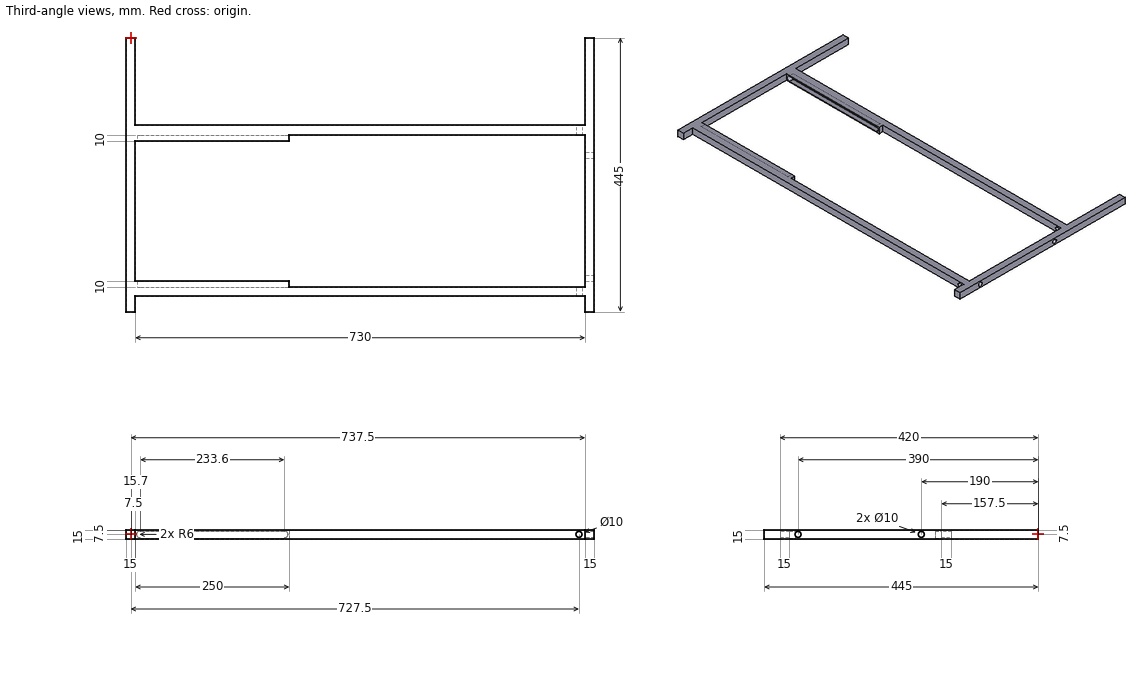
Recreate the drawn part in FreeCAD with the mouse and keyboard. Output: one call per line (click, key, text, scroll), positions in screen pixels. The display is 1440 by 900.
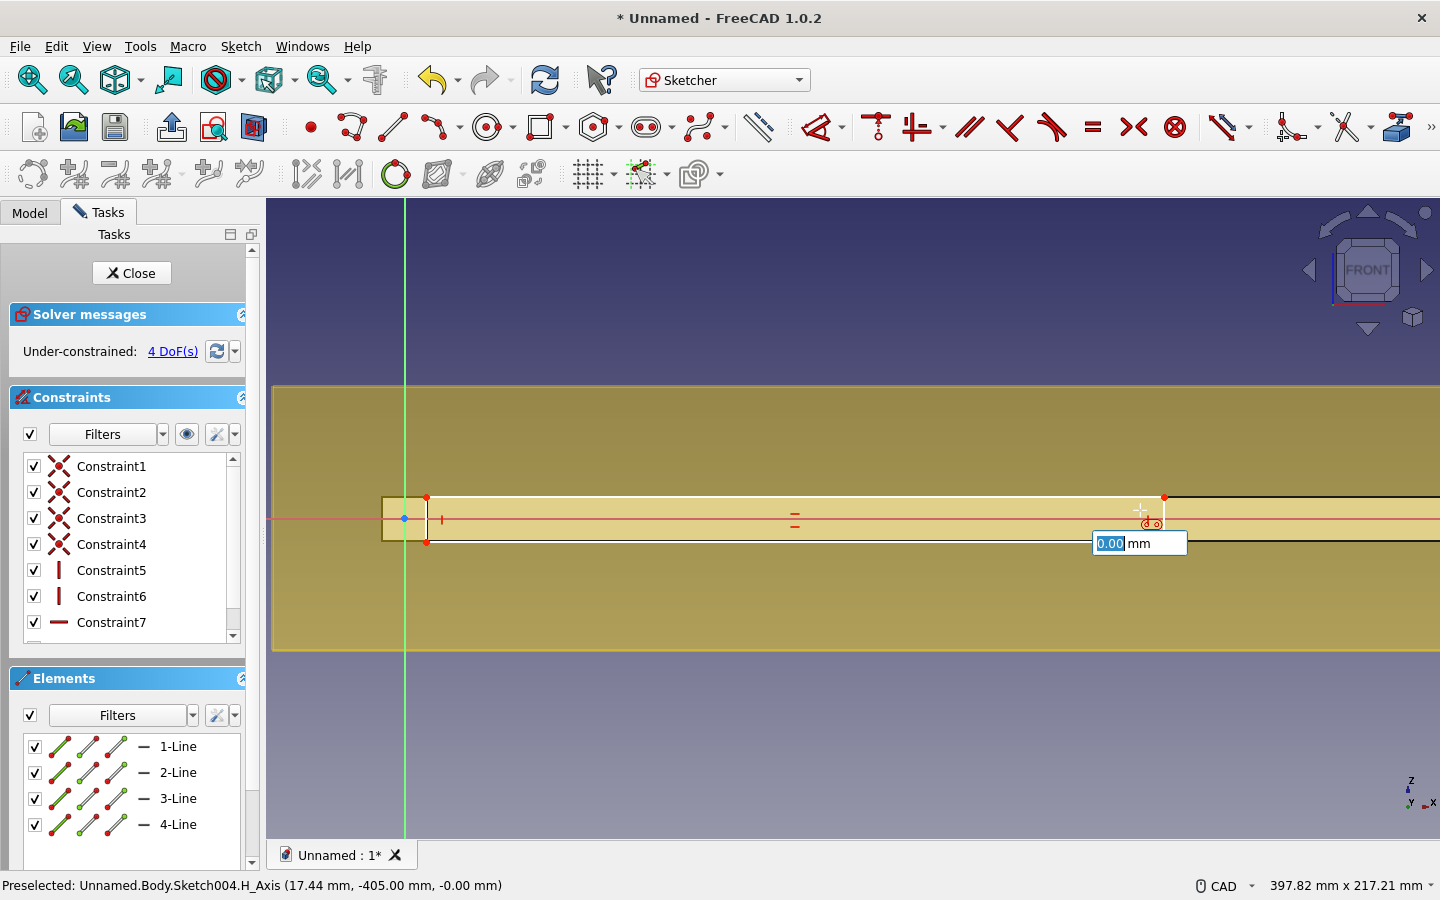
scroll(796, 501, up, 7)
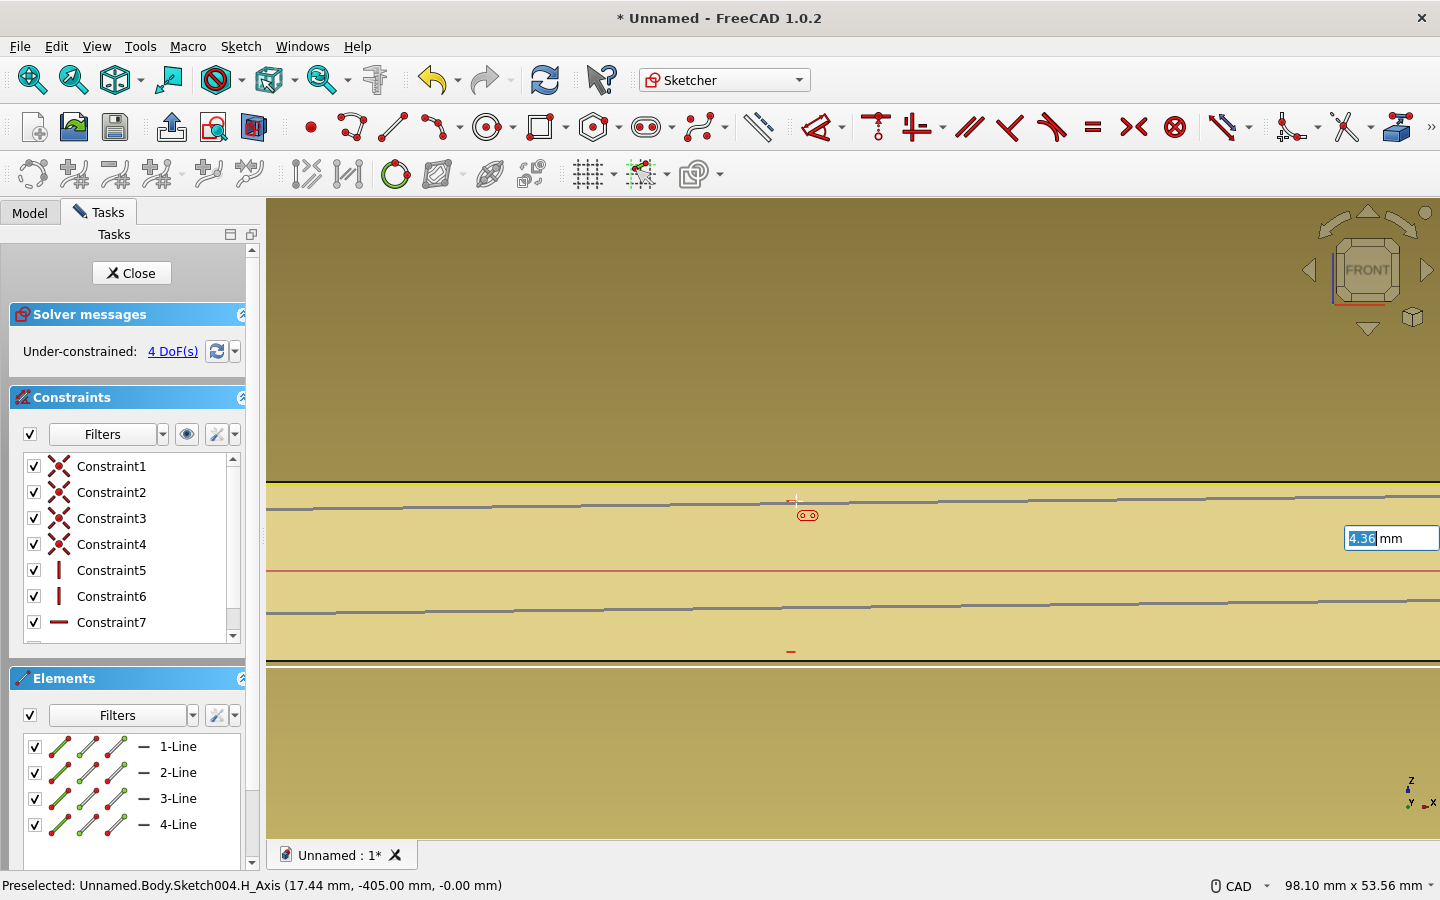
click(793, 500)
key(Escape)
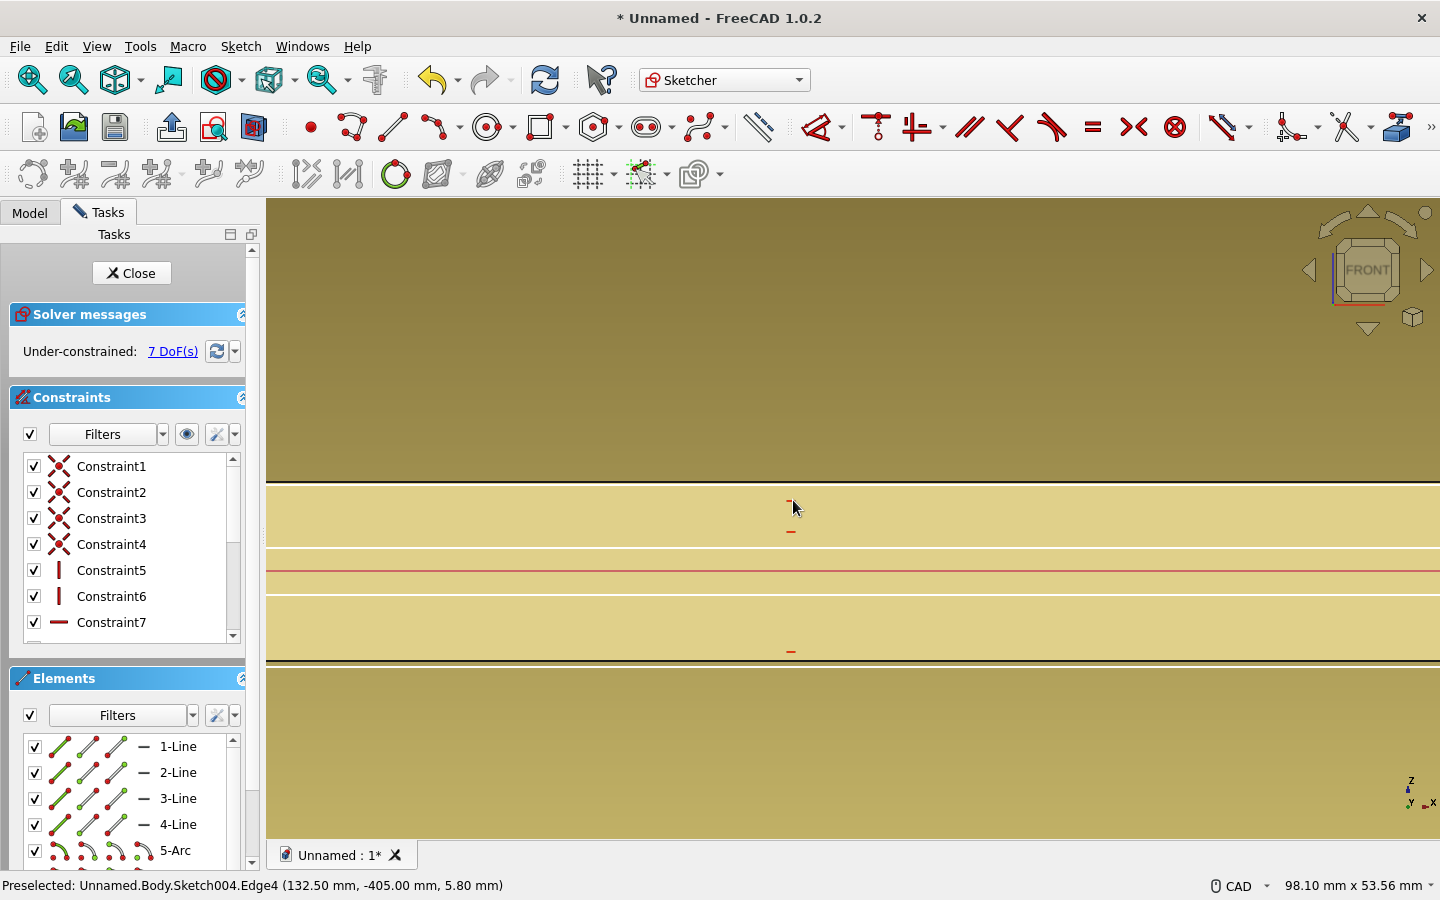
click(816, 128)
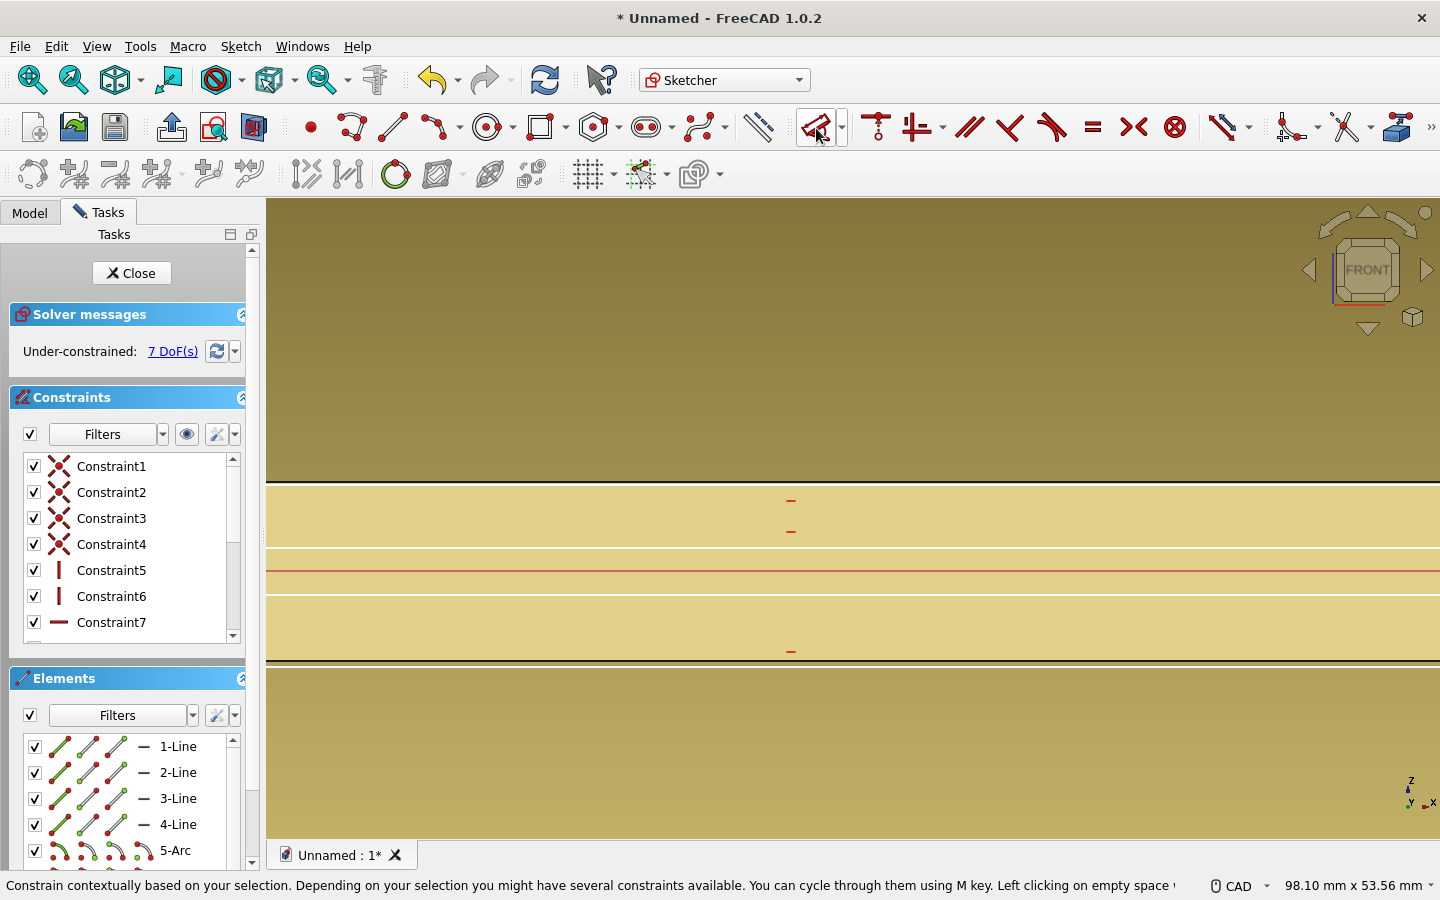
scroll(796, 501, down, 7)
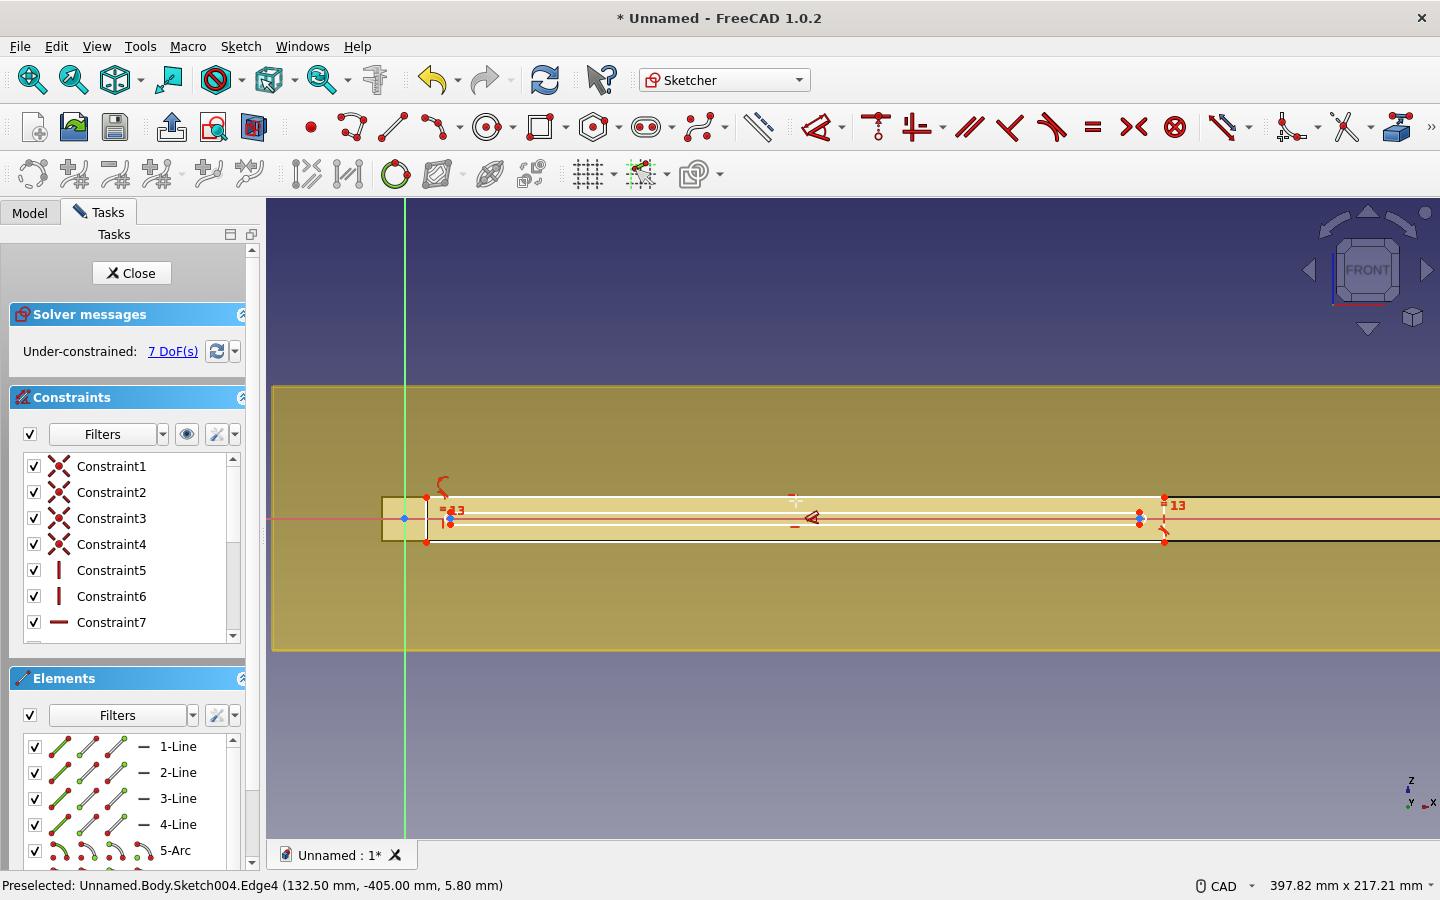
scroll(446, 515, up, 7)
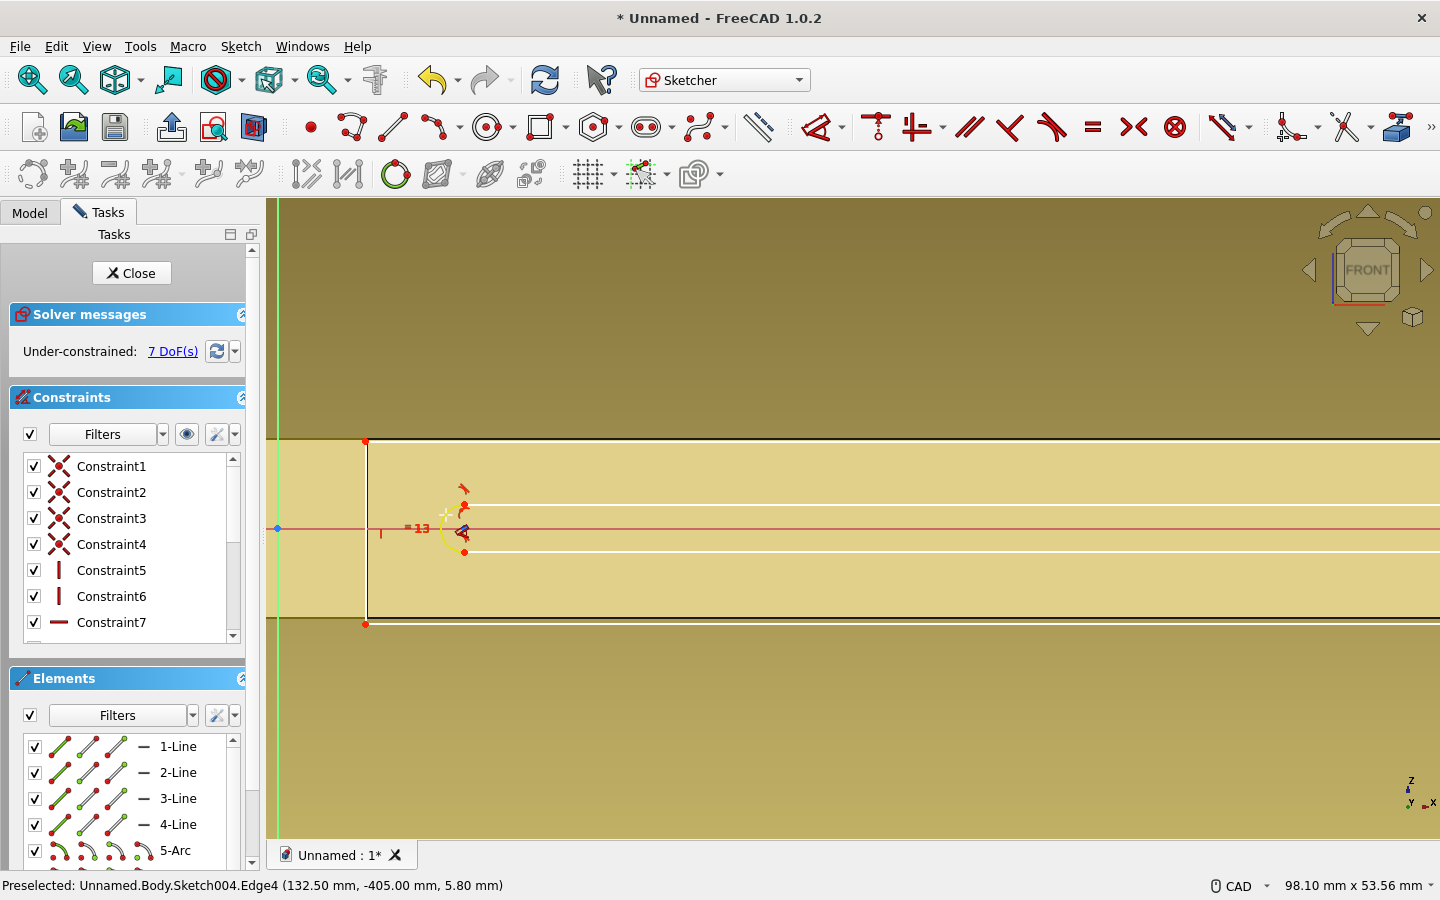
click(445, 515)
click(419, 497)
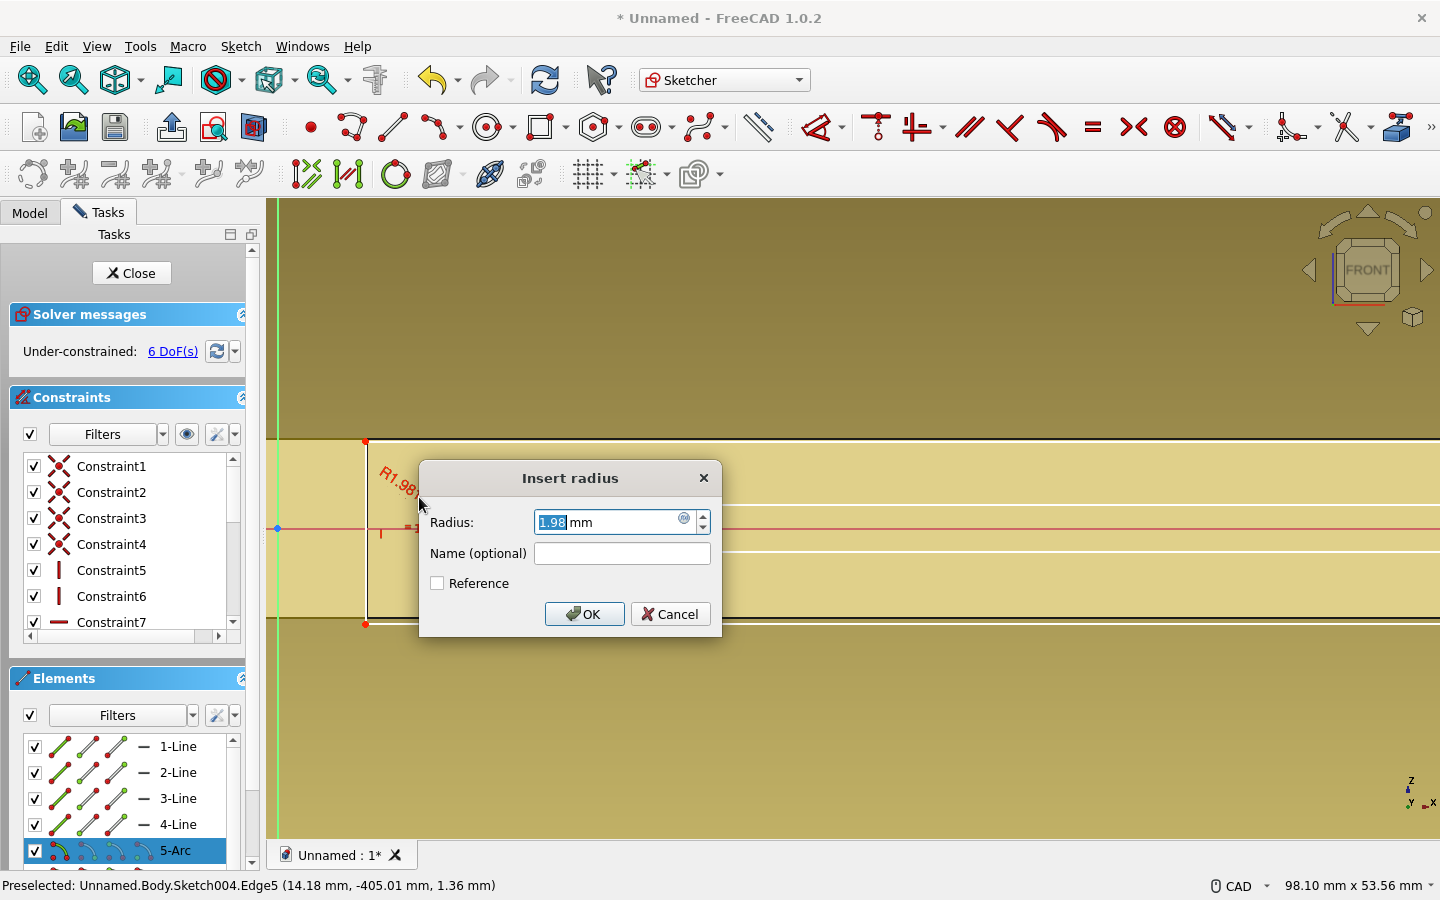
text(6)
key(Return)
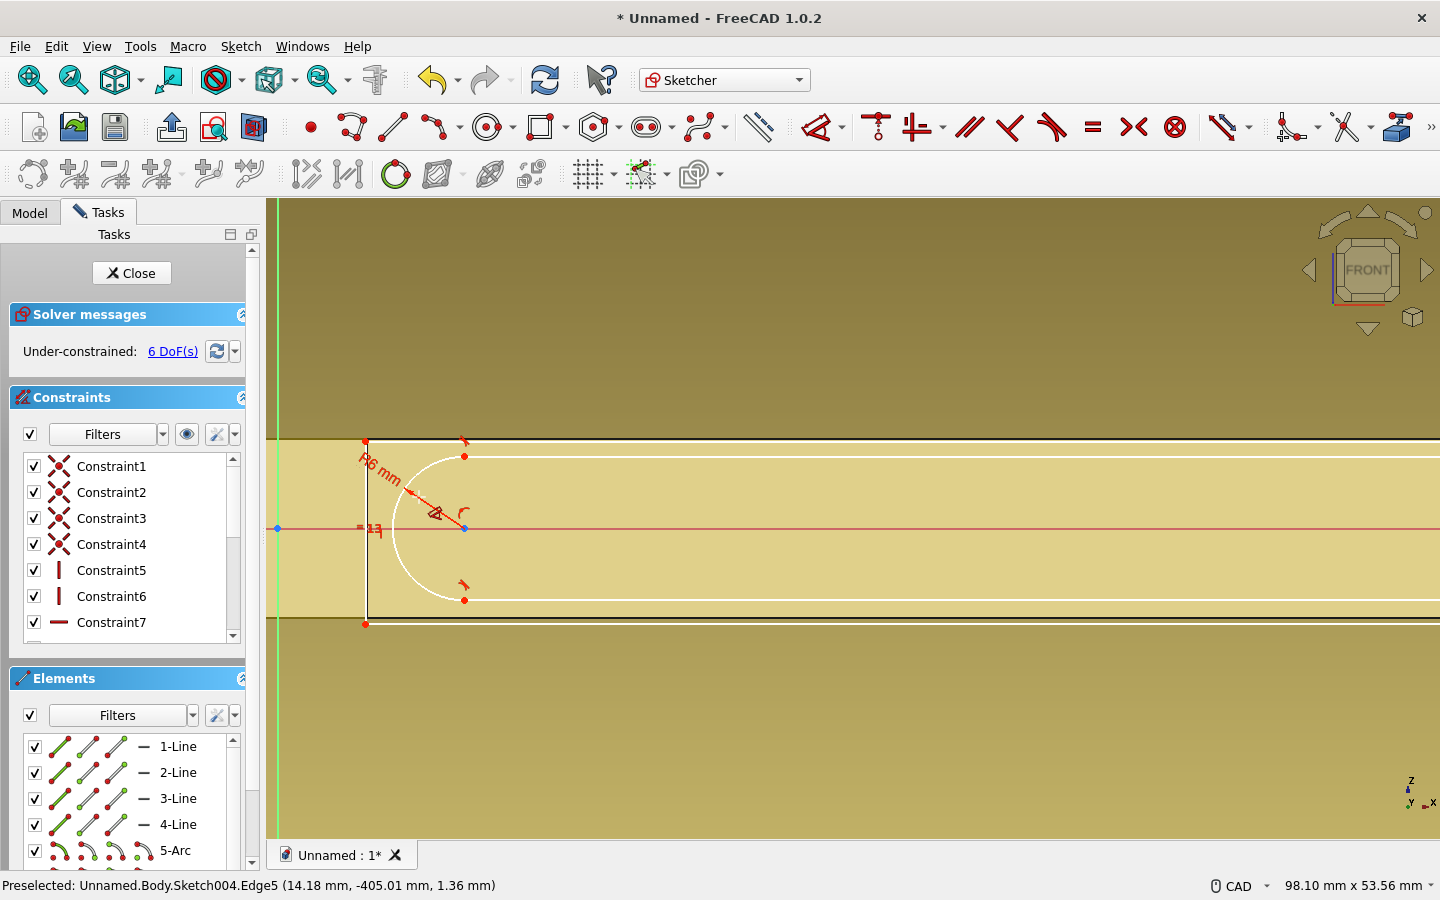
click(366, 497)
click(332, 491)